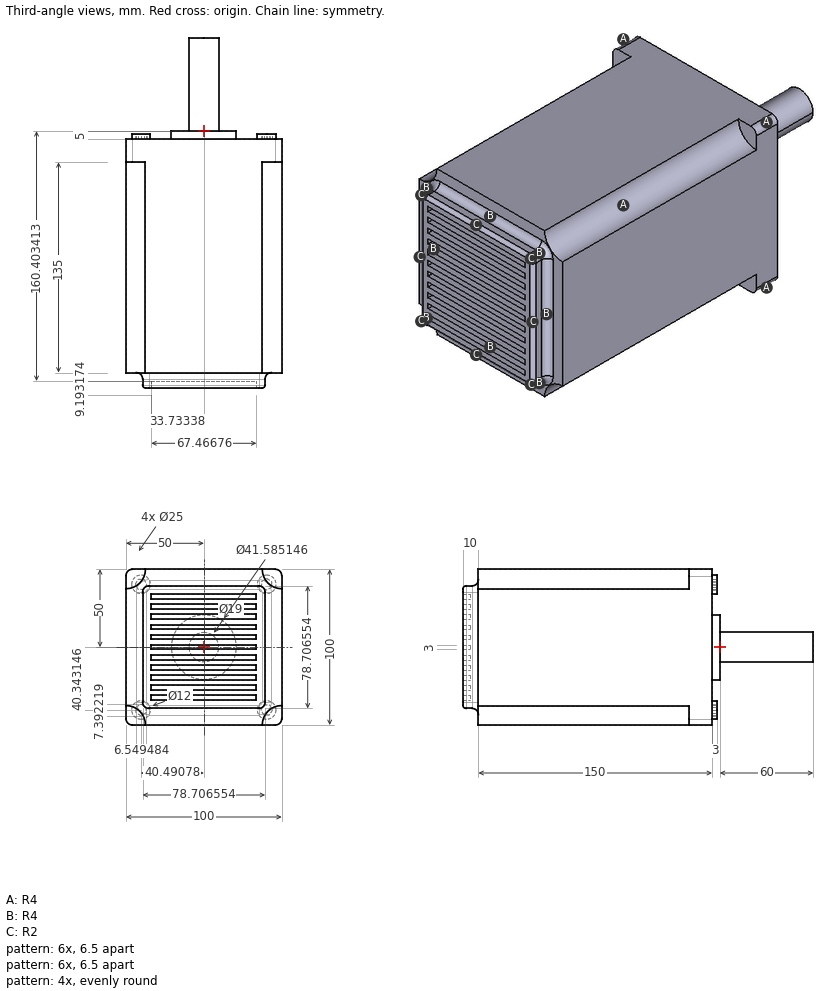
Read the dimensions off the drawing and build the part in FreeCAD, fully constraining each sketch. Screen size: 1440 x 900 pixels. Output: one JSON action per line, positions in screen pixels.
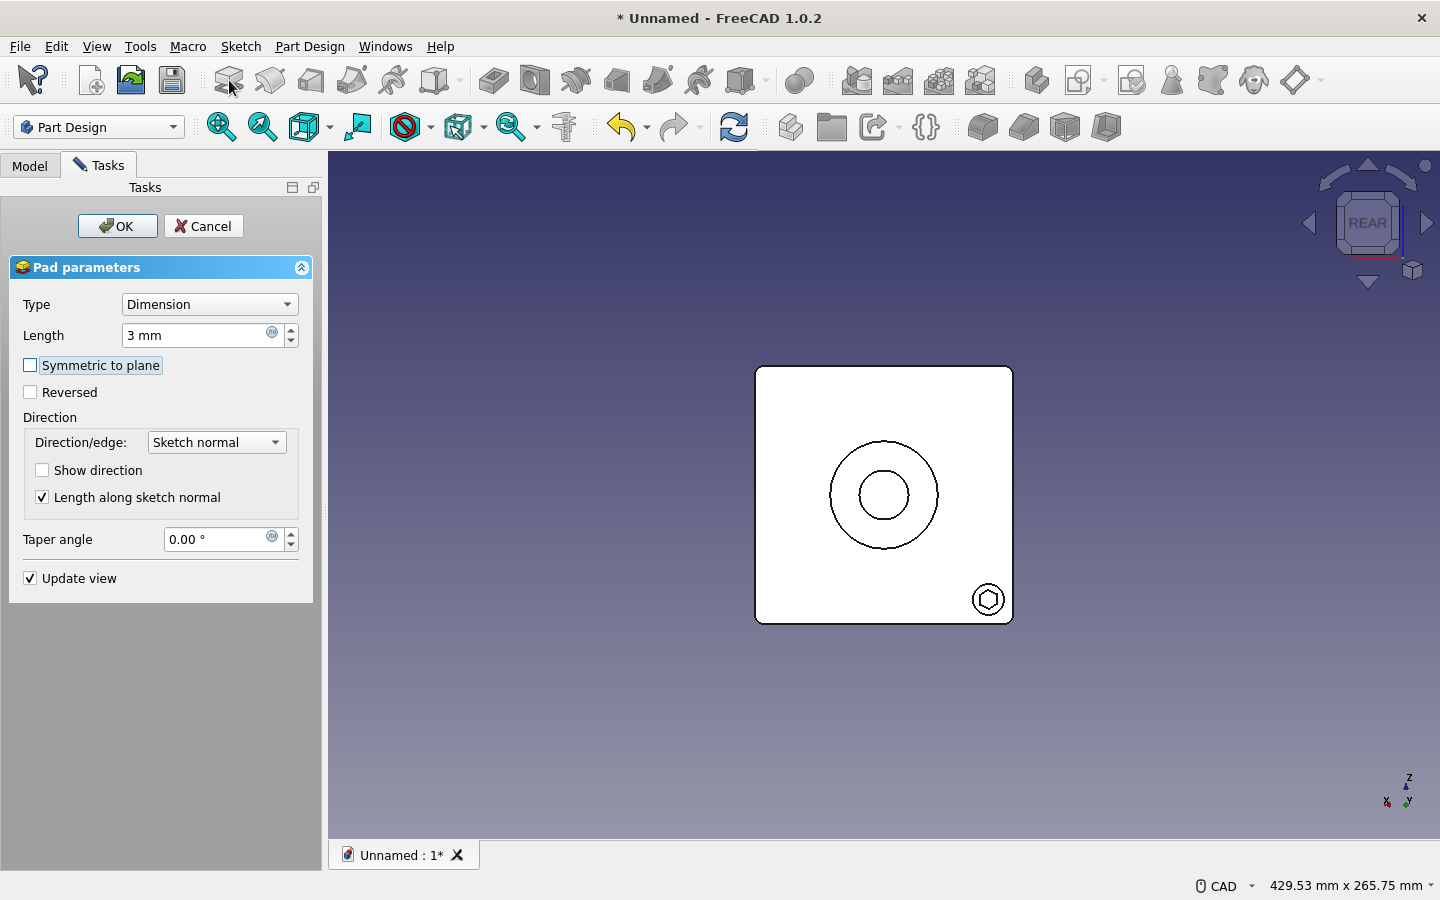
{"action": "left_click", "coordinate": [118, 226]}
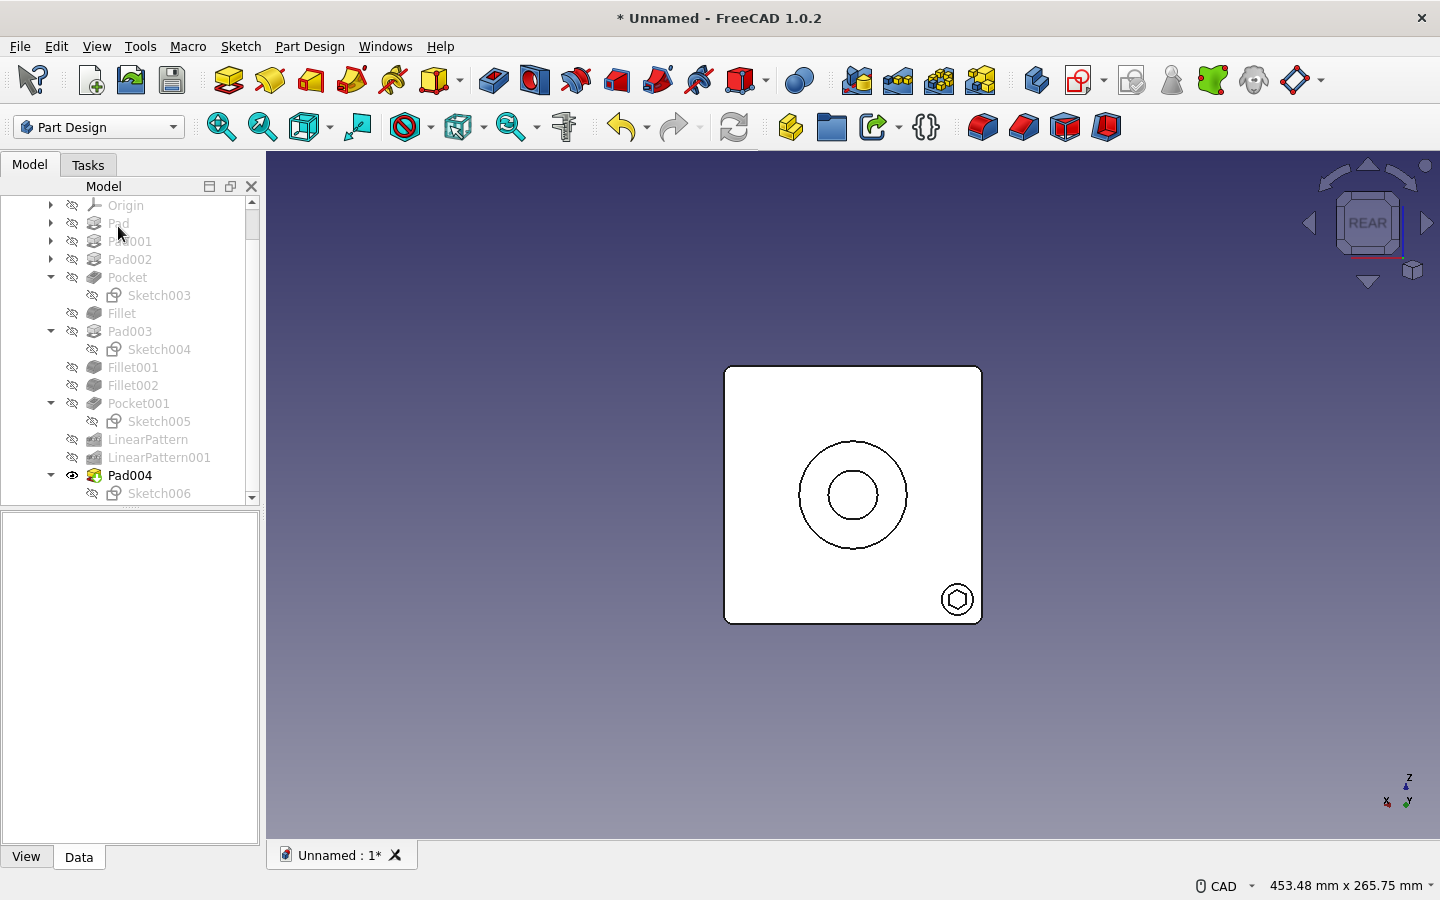
{"action": "left_click", "coordinate": [222, 128]}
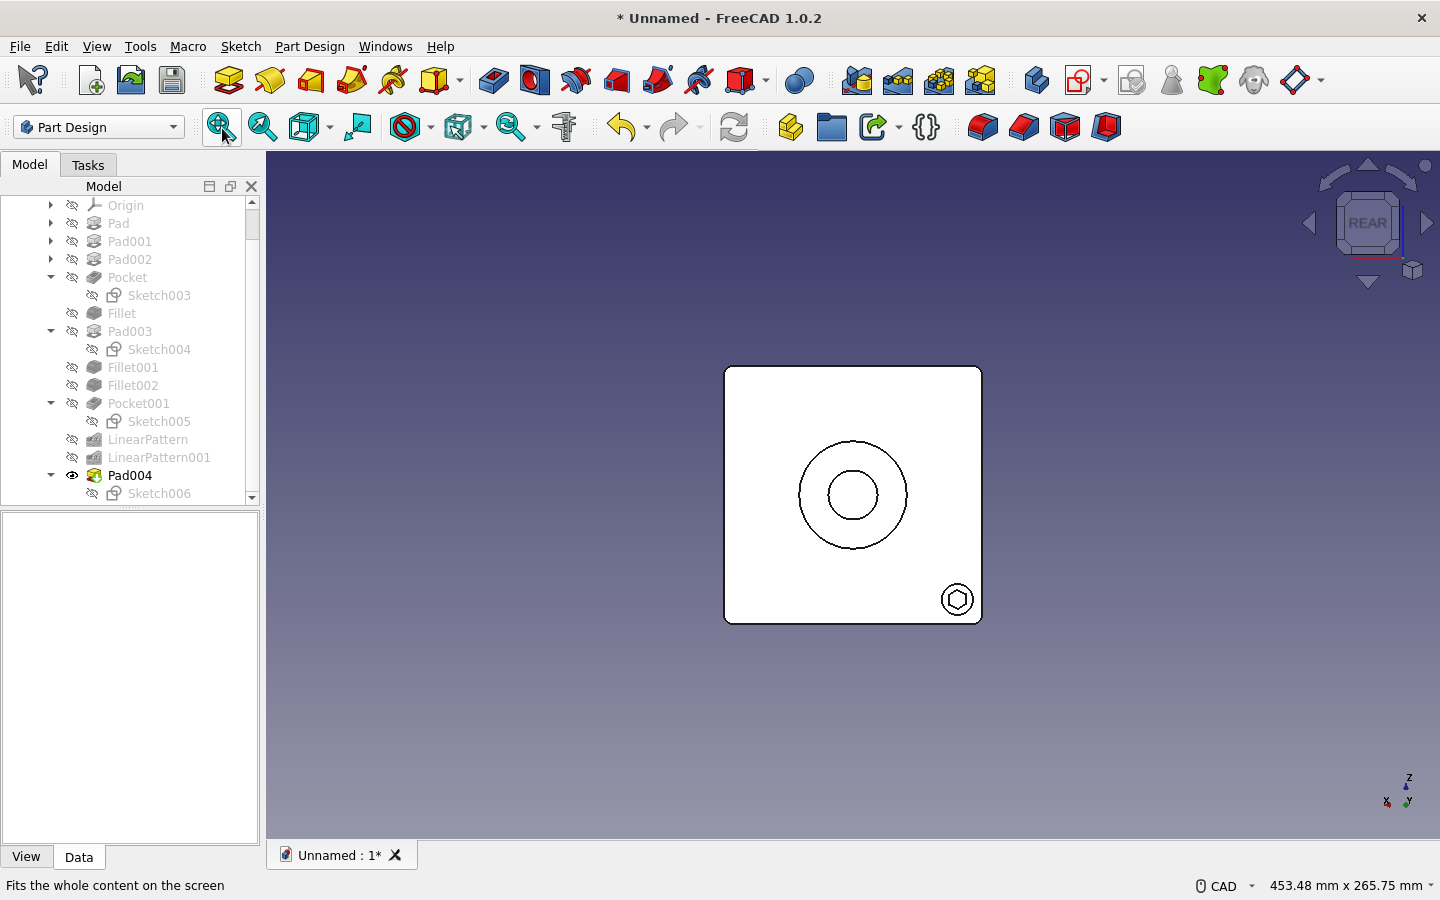
{"action": "left_click", "coordinate": [117, 475]}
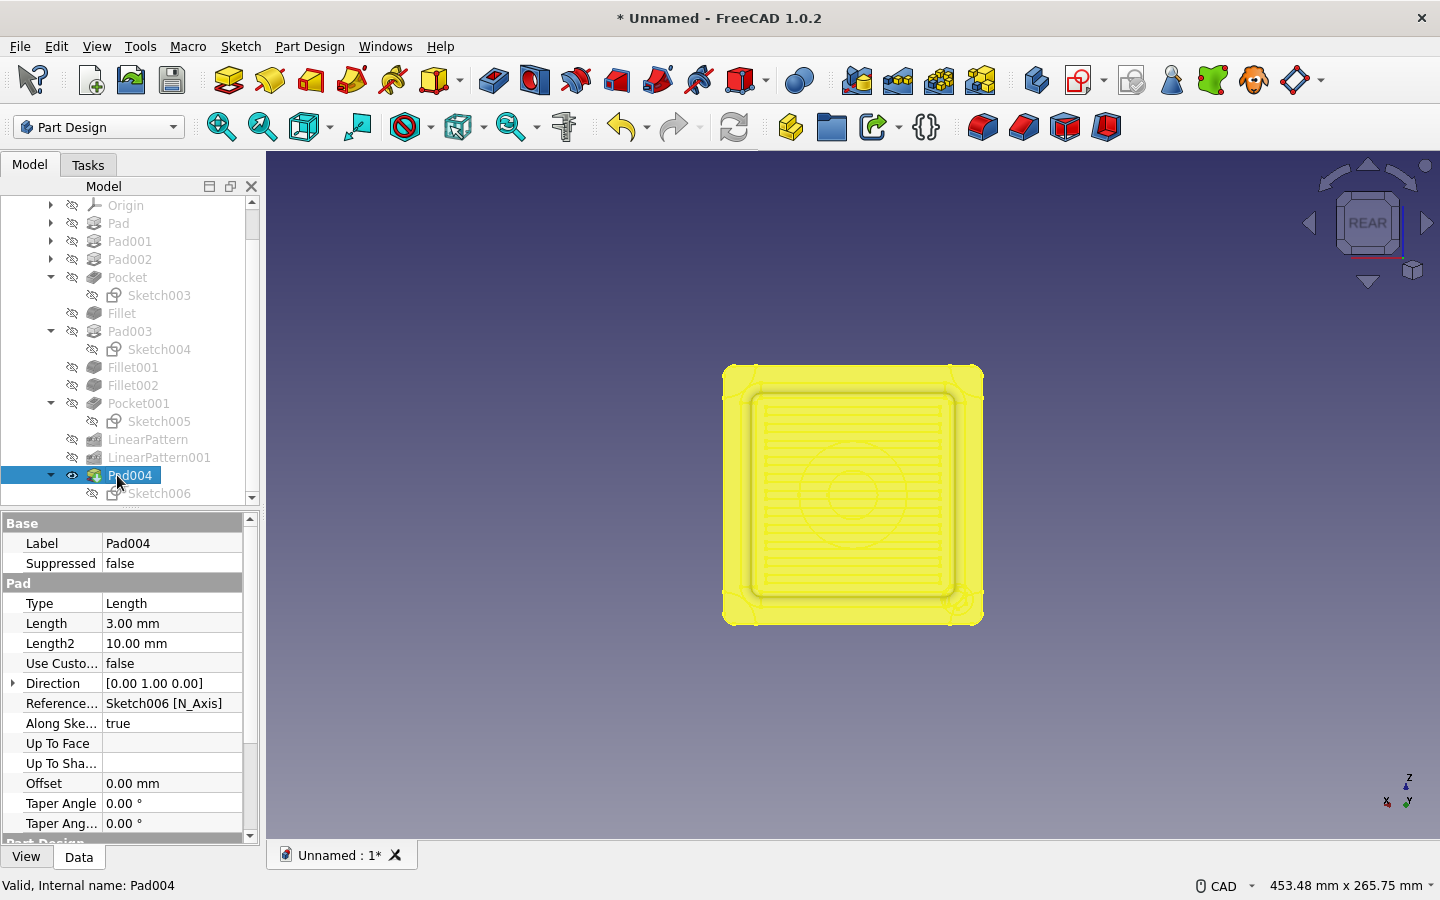
{"action": "left_click", "coordinate": [939, 80]}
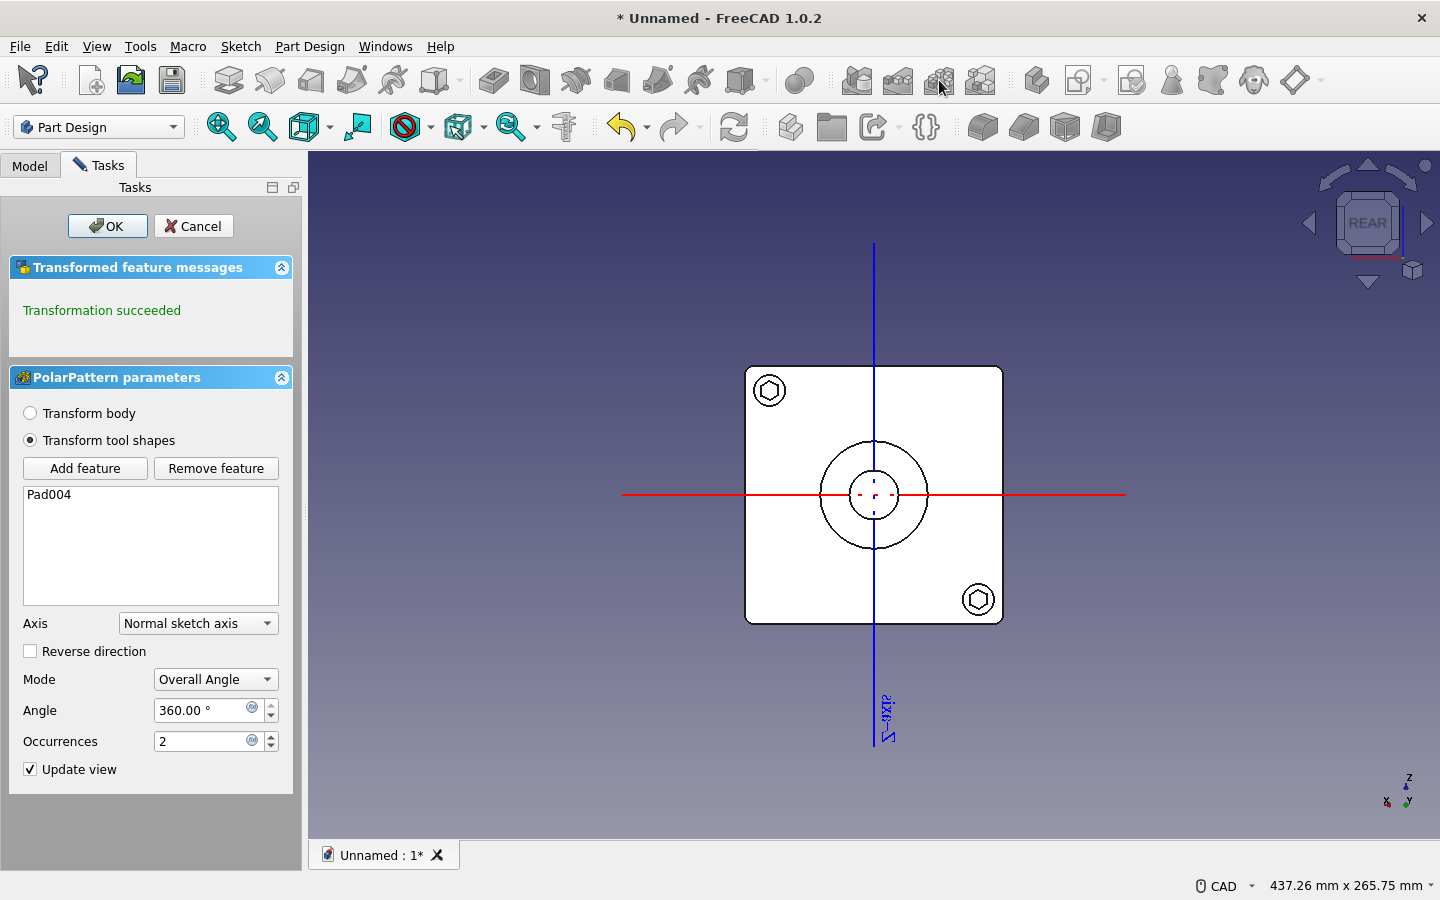
{"action": "left_click", "coordinate": [199, 624]}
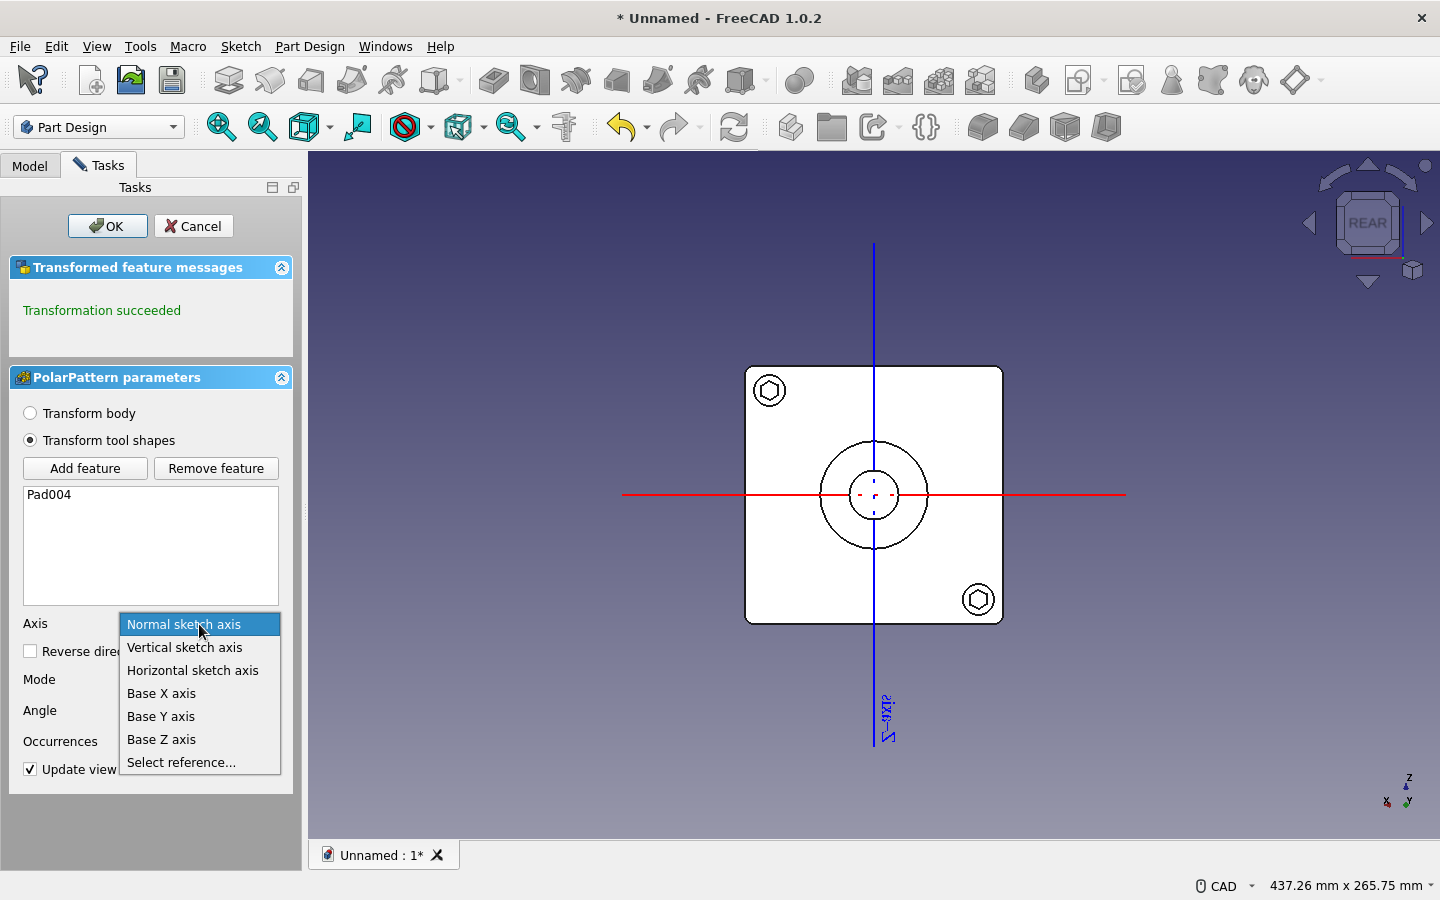
{"action": "left_click", "coordinate": [198, 716]}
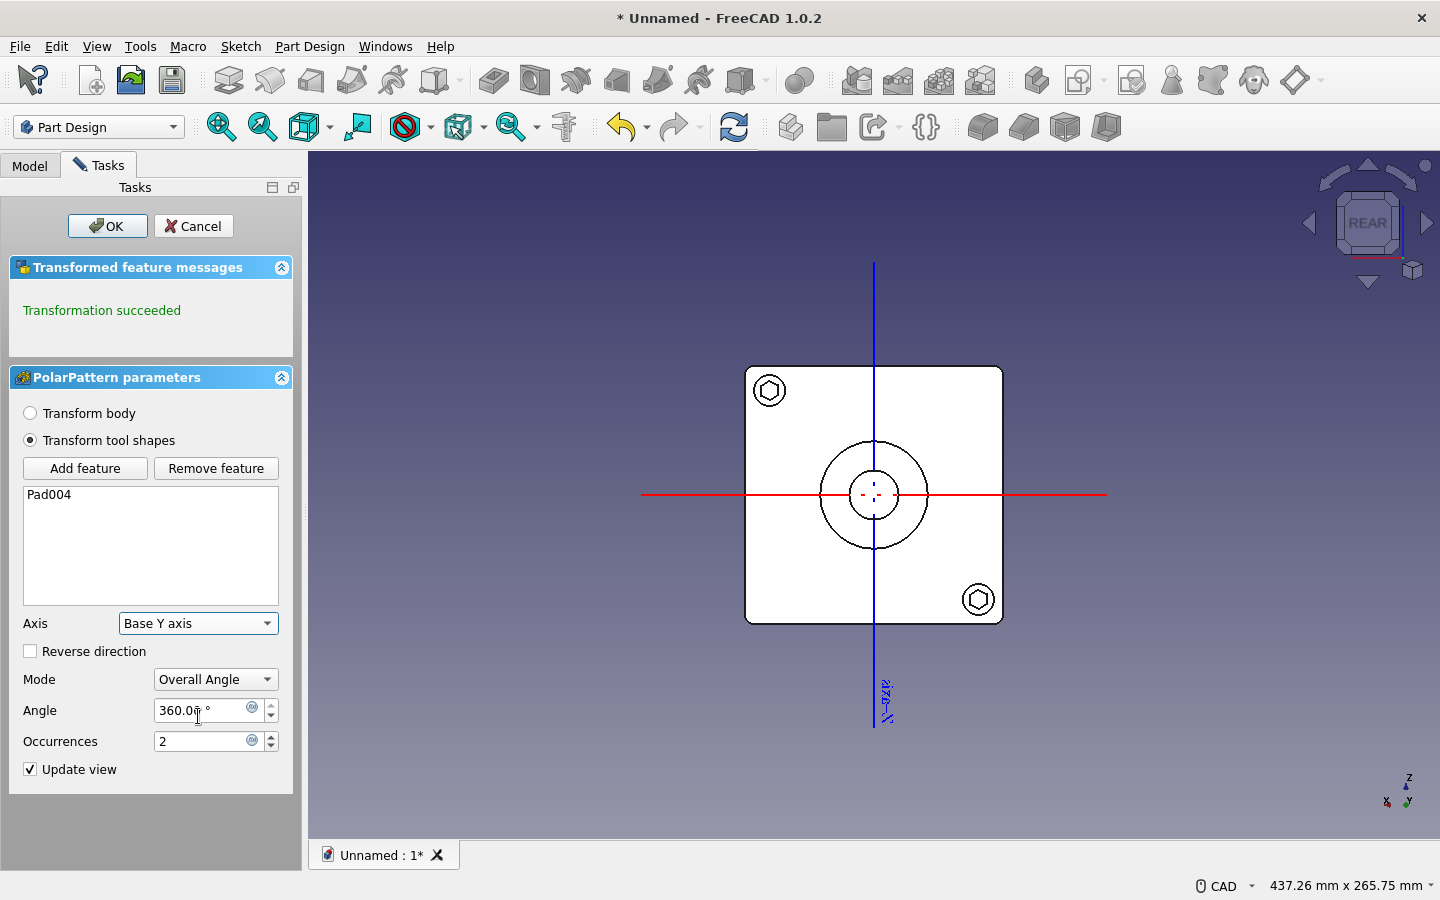
{"action": "triple_click", "coordinate": [210, 742]}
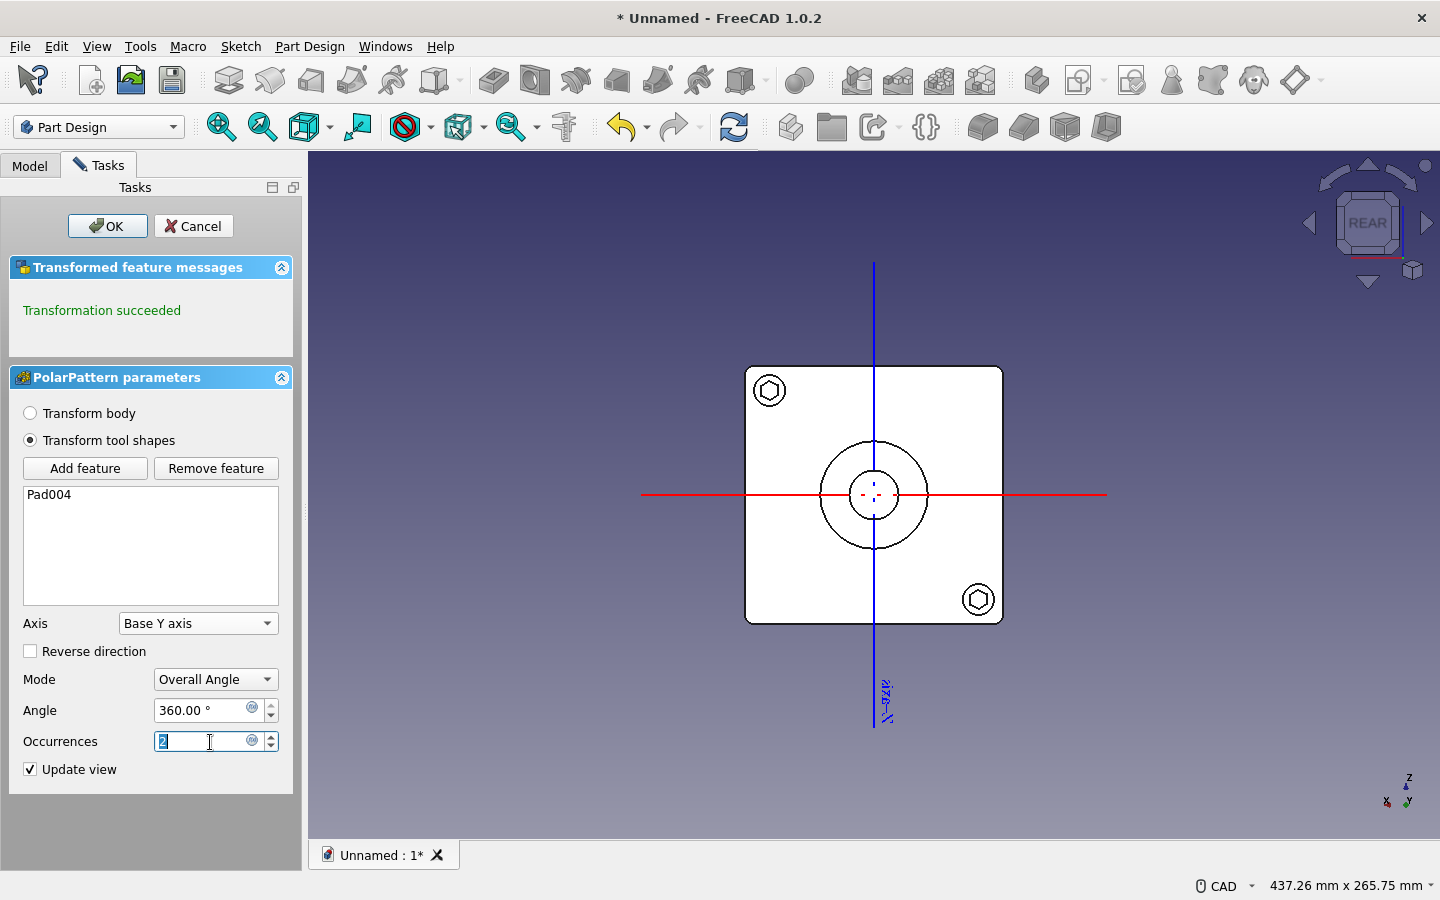
{"action": "type", "text": "4"}
{"action": "key", "text": "Tab"}